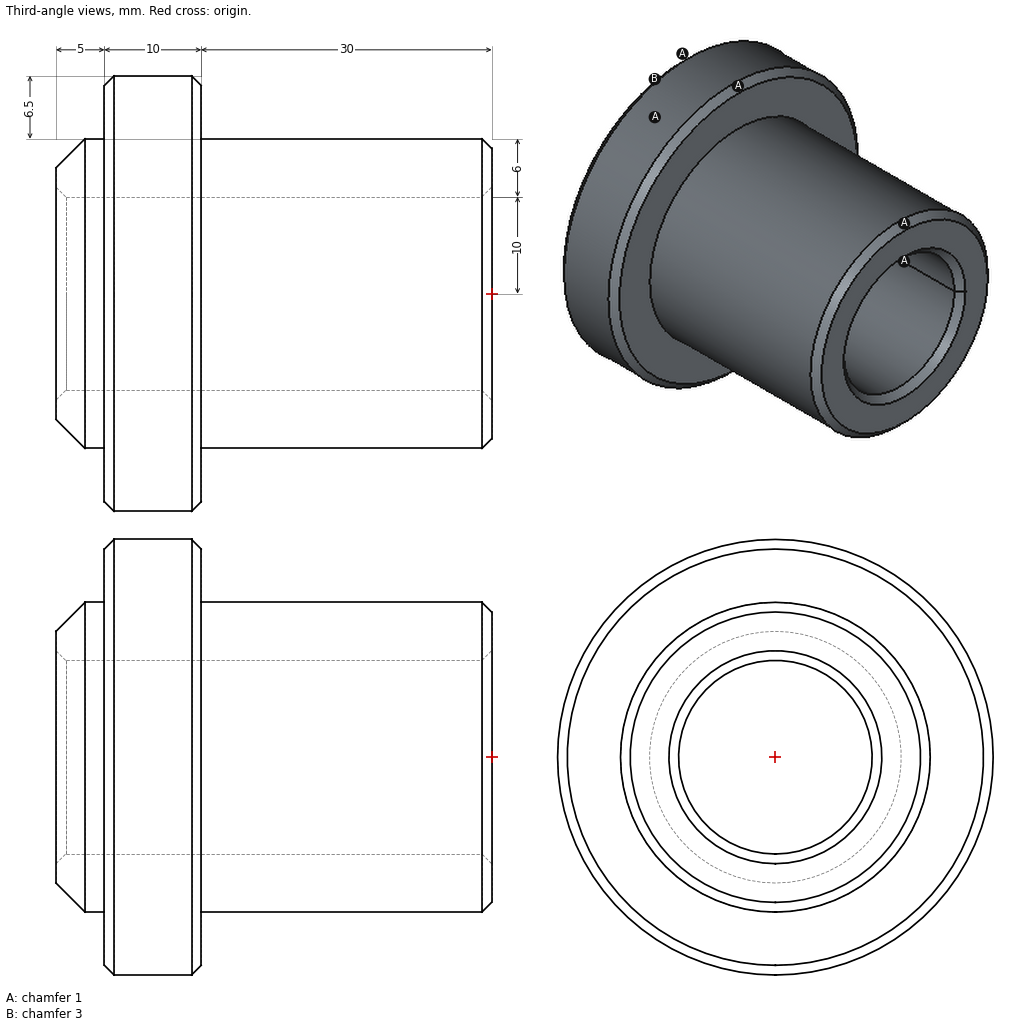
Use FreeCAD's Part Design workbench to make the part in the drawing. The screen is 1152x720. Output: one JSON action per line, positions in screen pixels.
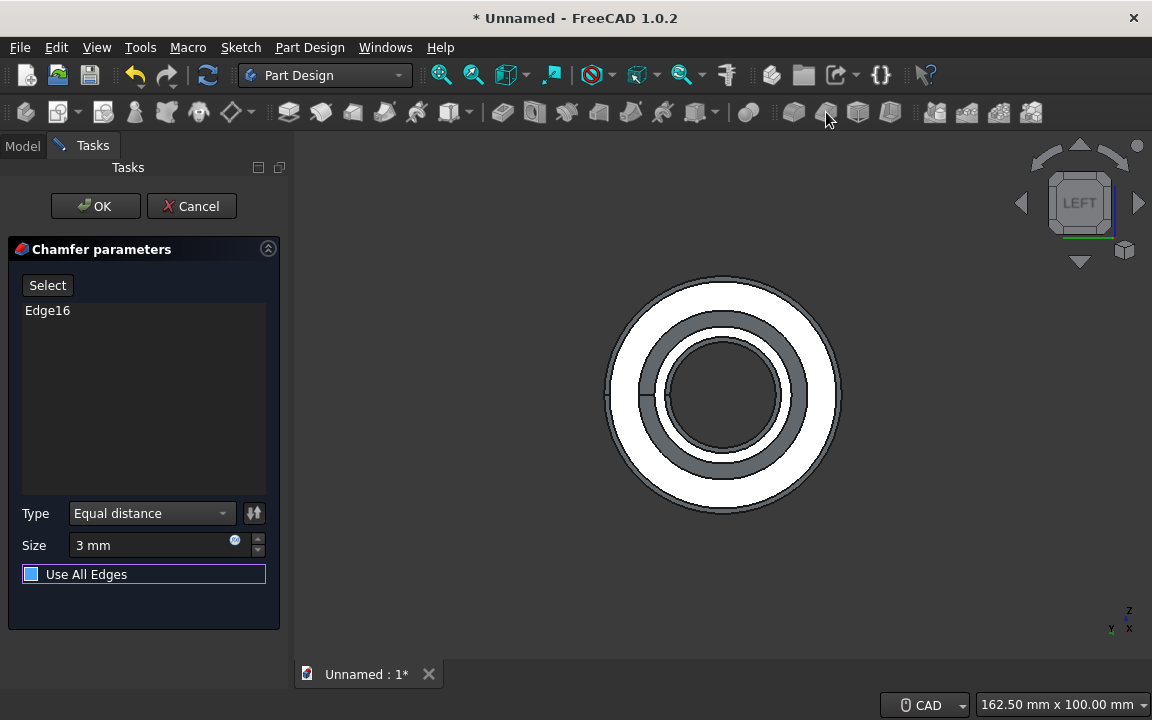
{"action": "left_click", "coordinate": [96, 206]}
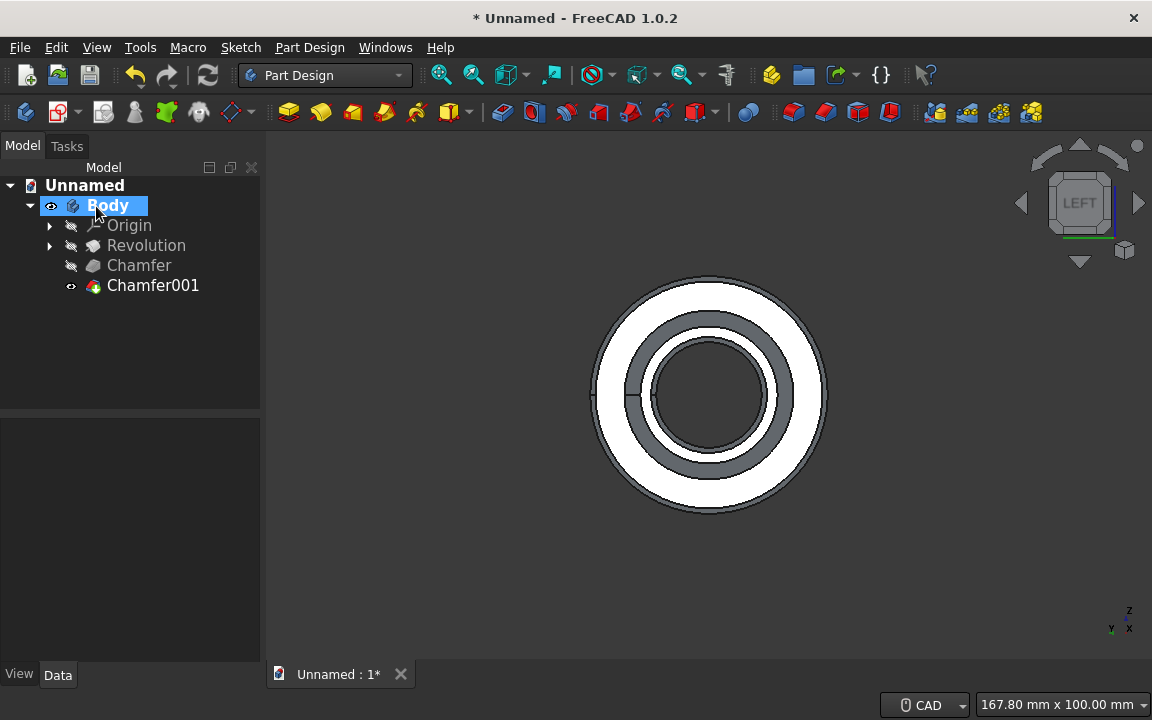
{"action": "key", "text": "0"}